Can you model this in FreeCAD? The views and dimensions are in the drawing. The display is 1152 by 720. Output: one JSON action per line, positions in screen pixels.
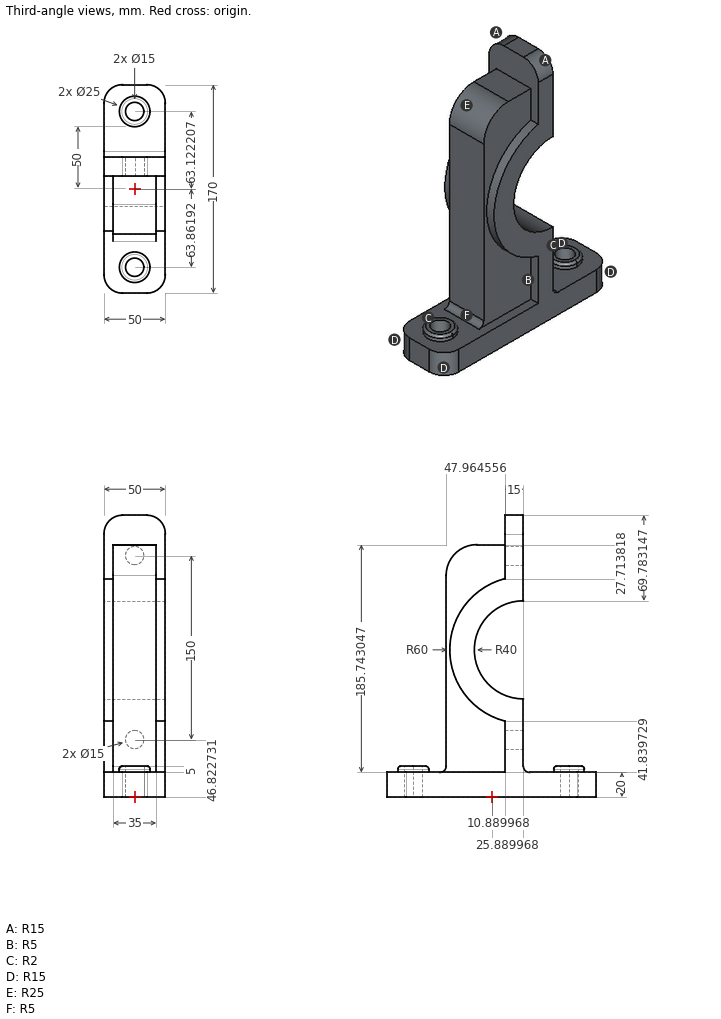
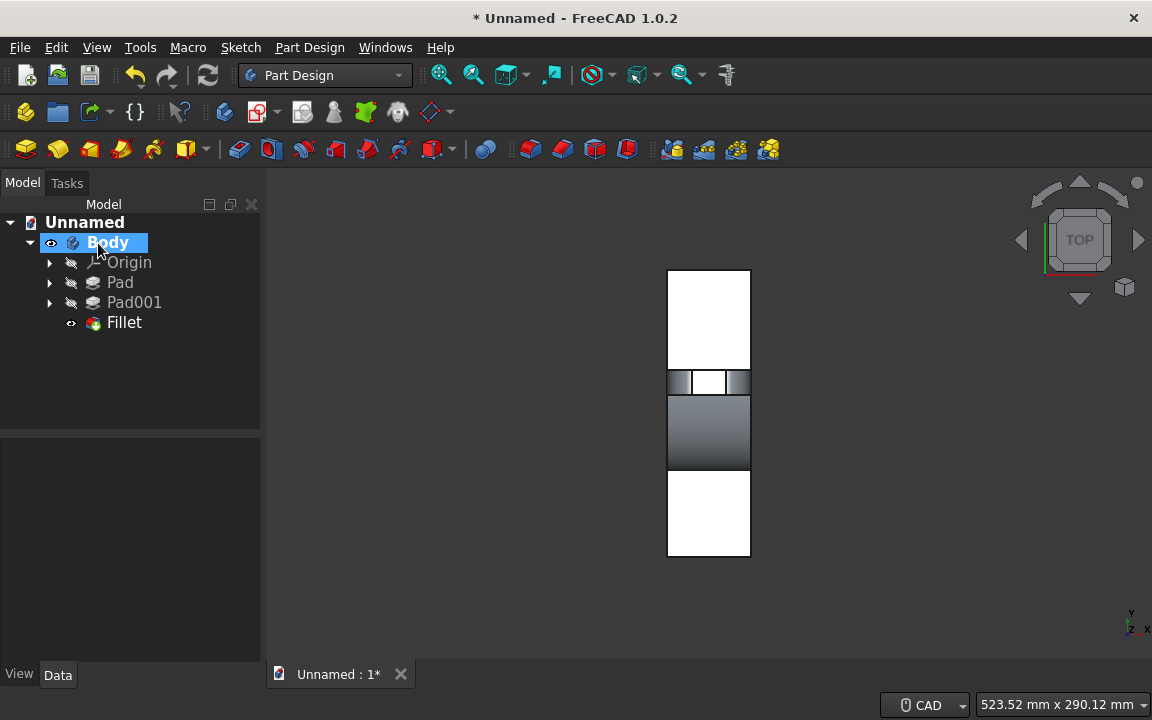
{"action": "key", "text": "0"}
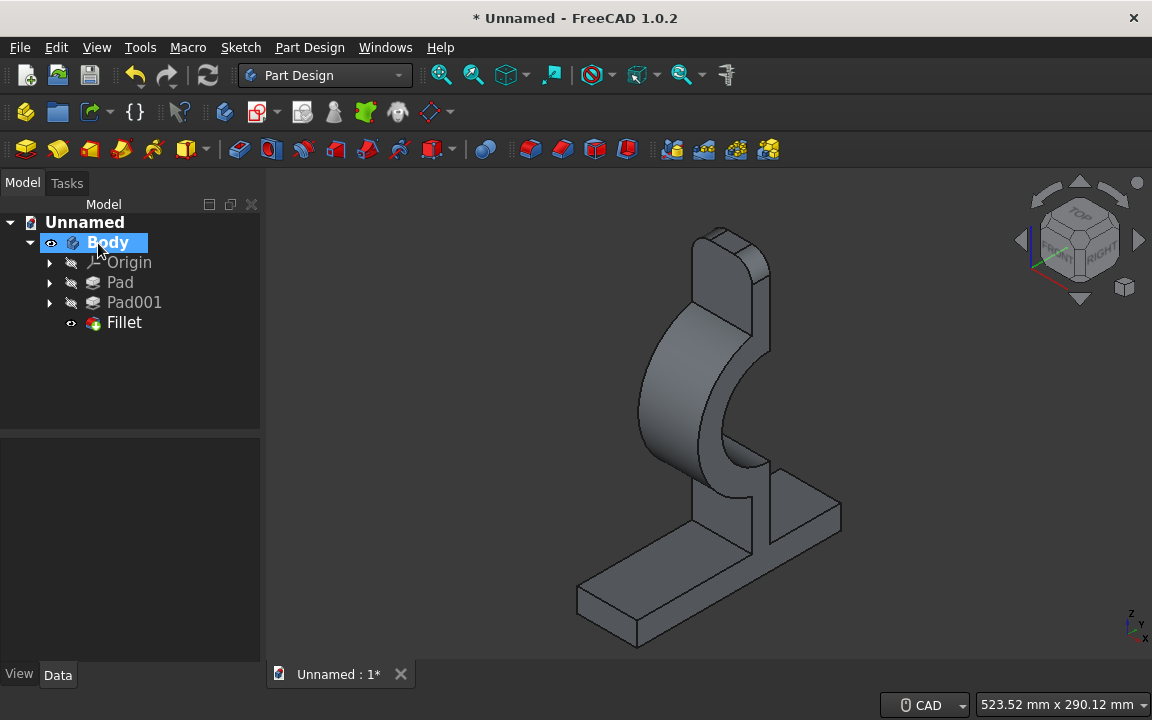
{"action": "key", "text": "2"}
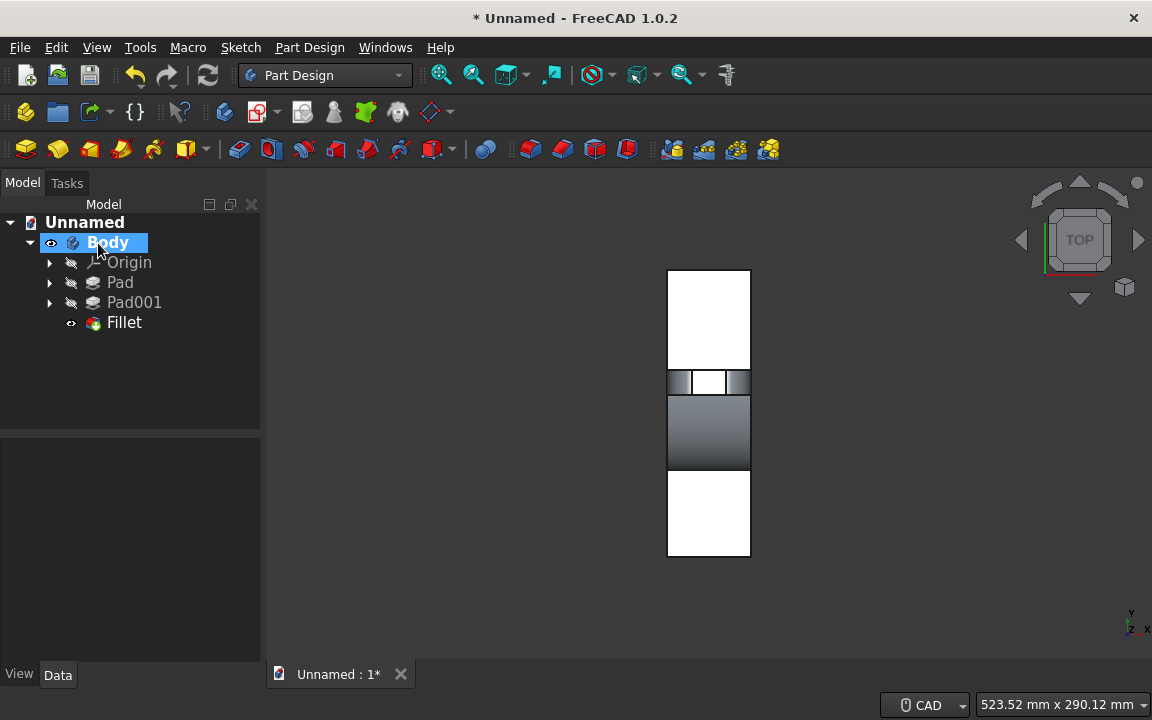
{"action": "key", "text": "1"}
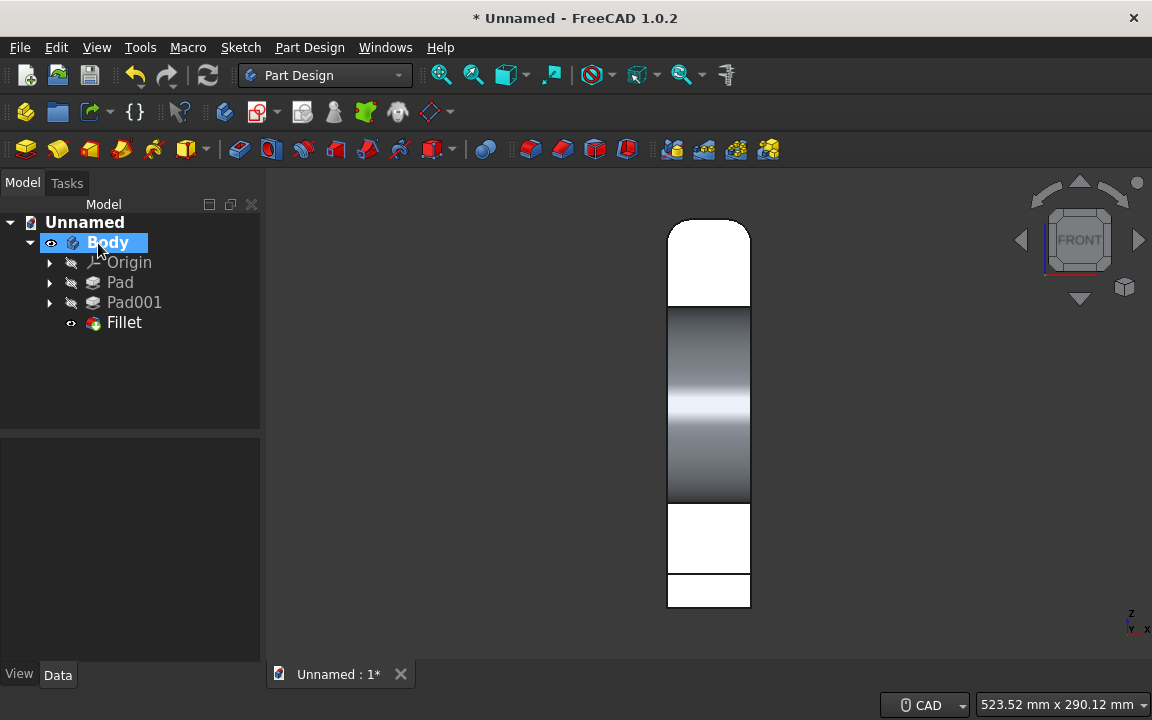
{"action": "key", "text": "3"}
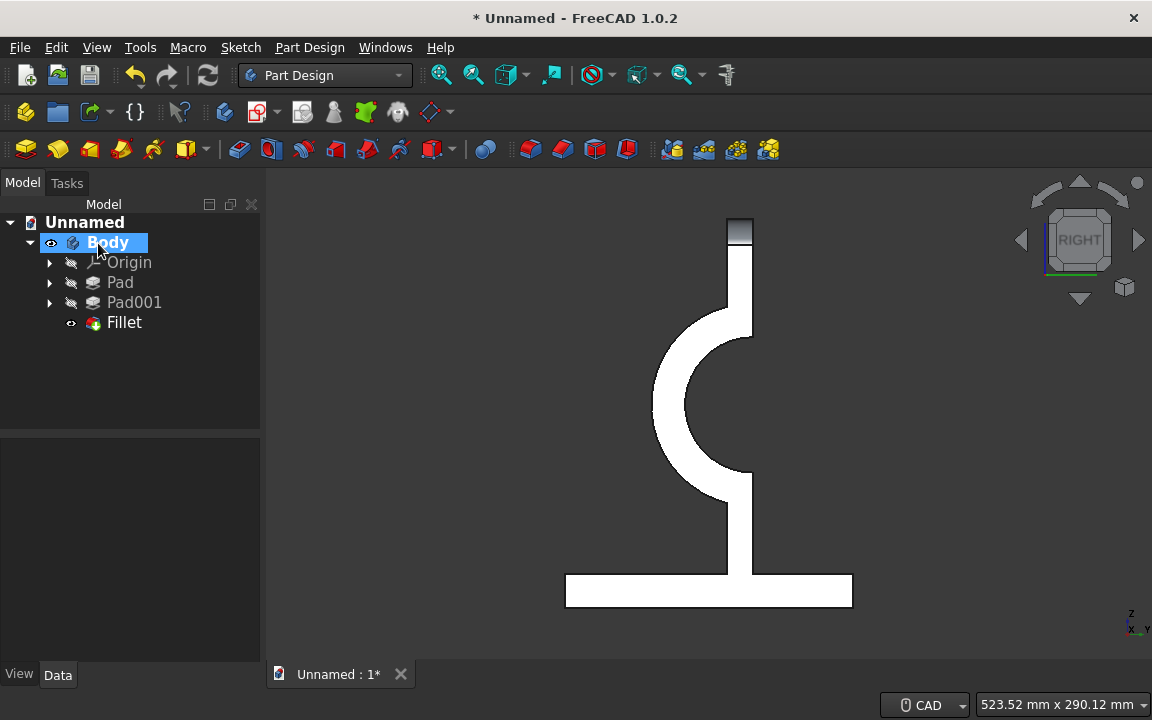
{"action": "key", "text": "5"}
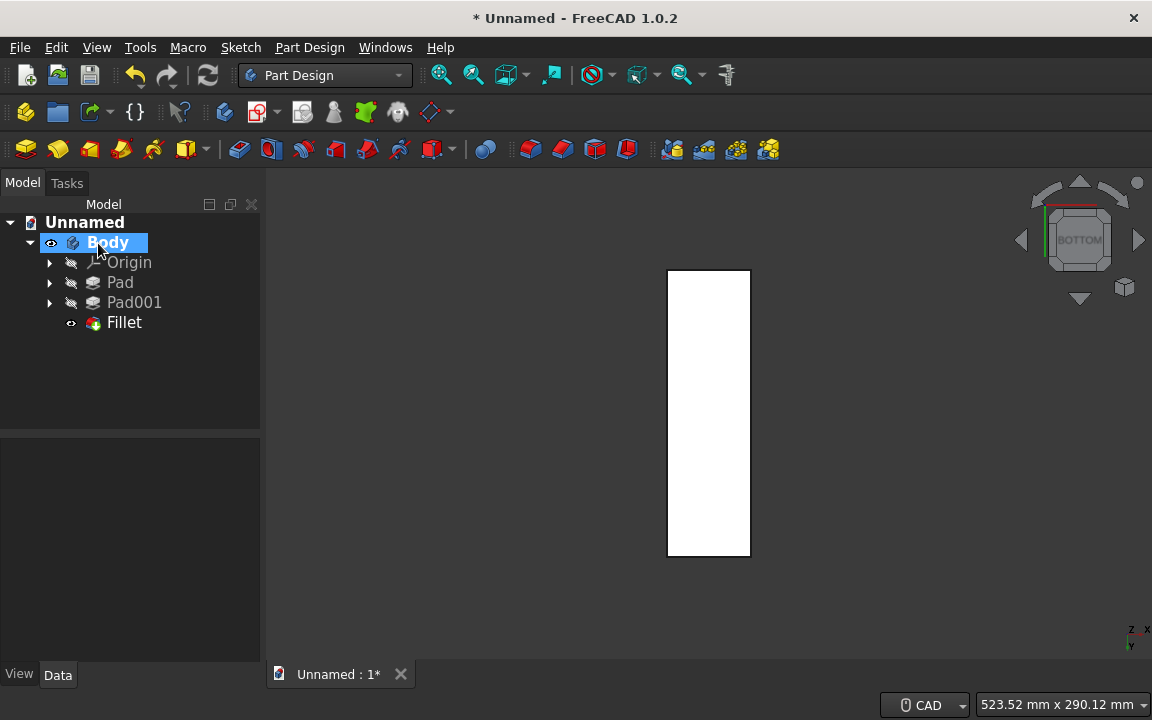
{"action": "key", "text": "4"}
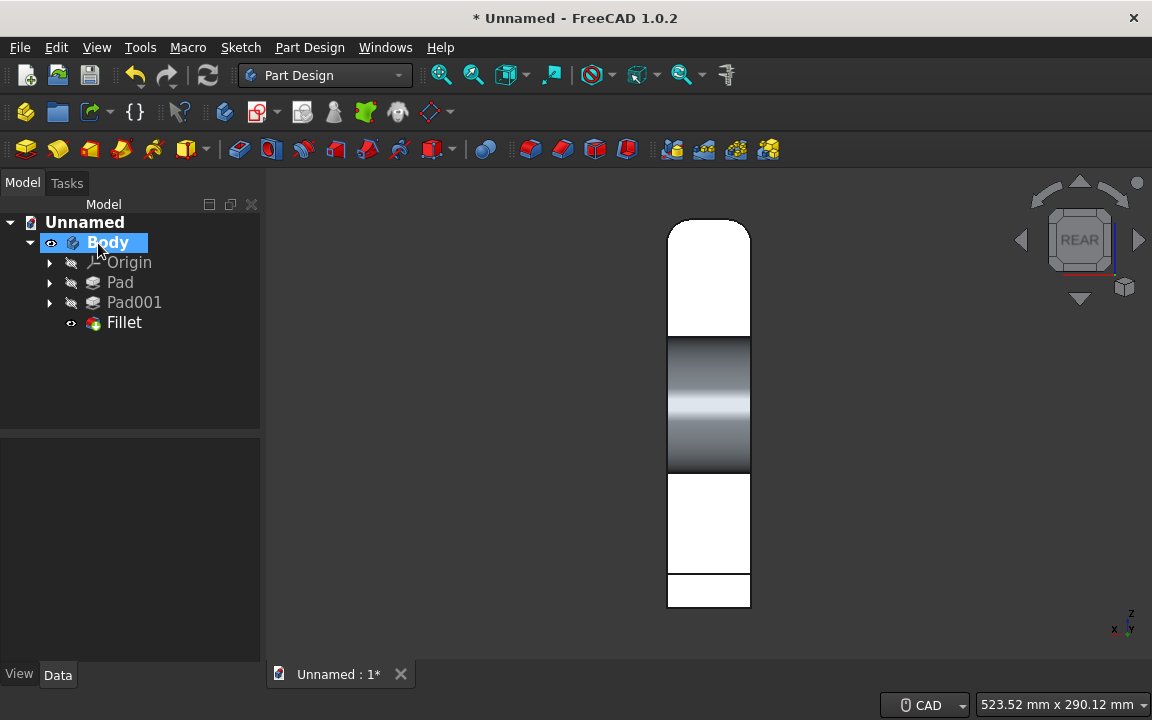
{"action": "key", "text": "6"}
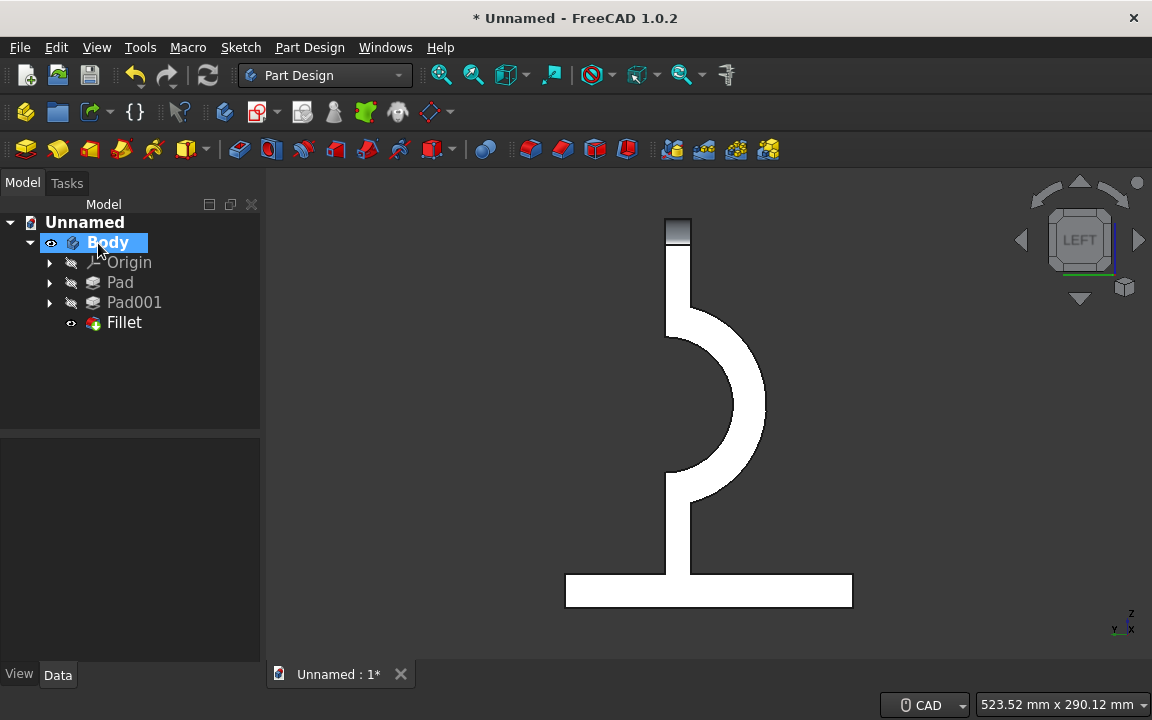
{"action": "key", "text": "v 3"}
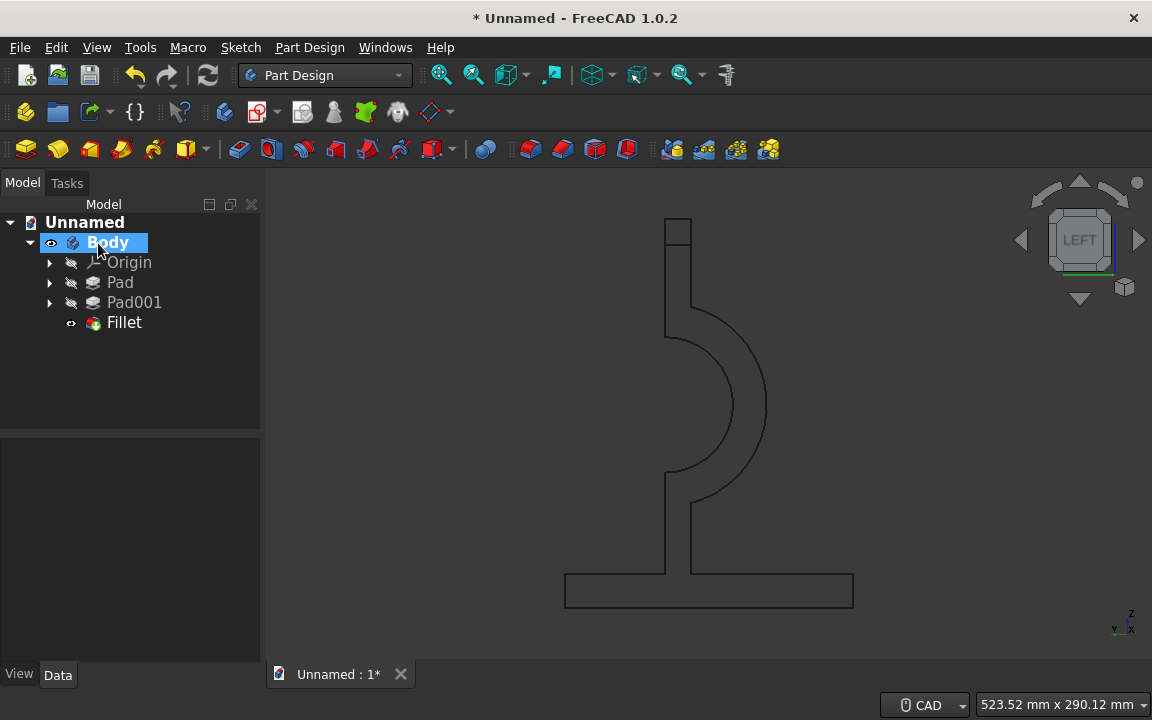
{"action": "key", "text": "0"}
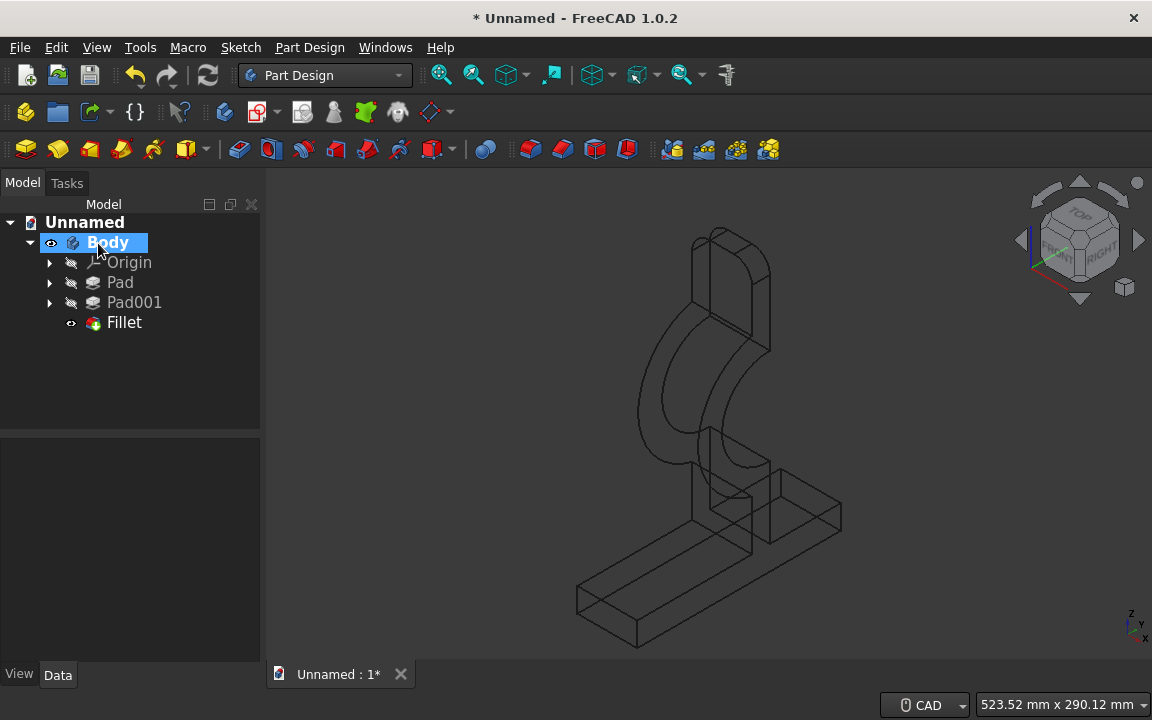
{"action": "left_click", "coordinate": [740, 526]}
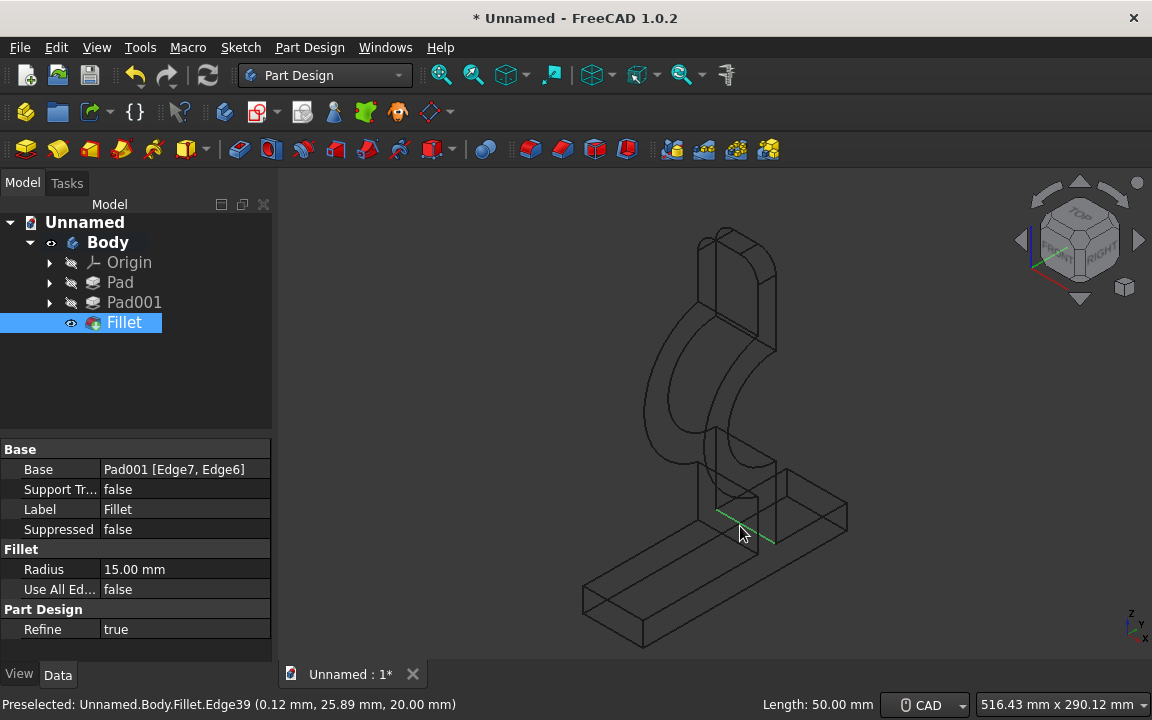
{"action": "key", "text": "v 1"}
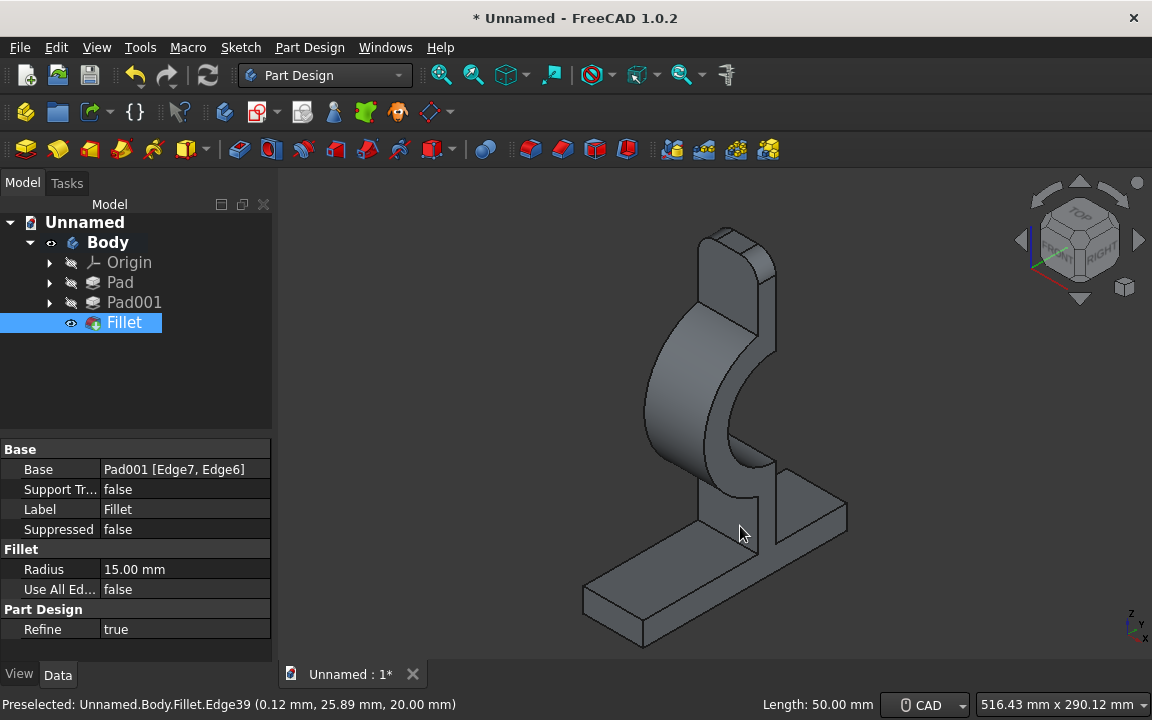
{"action": "left_click", "coordinate": [532, 150]}